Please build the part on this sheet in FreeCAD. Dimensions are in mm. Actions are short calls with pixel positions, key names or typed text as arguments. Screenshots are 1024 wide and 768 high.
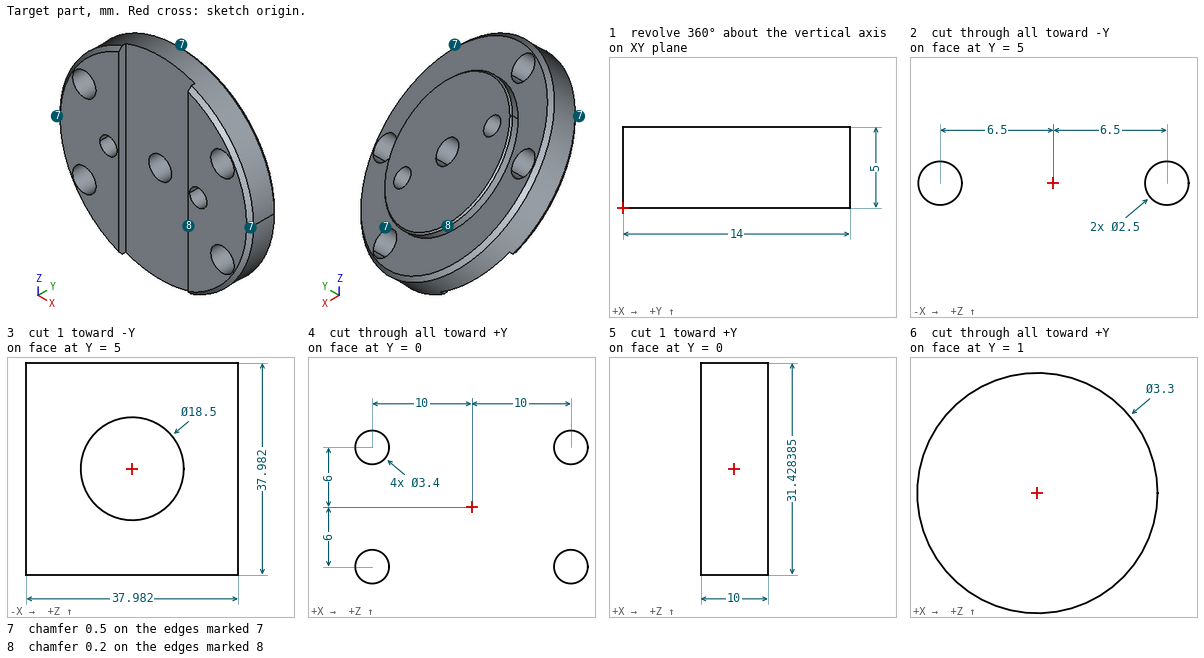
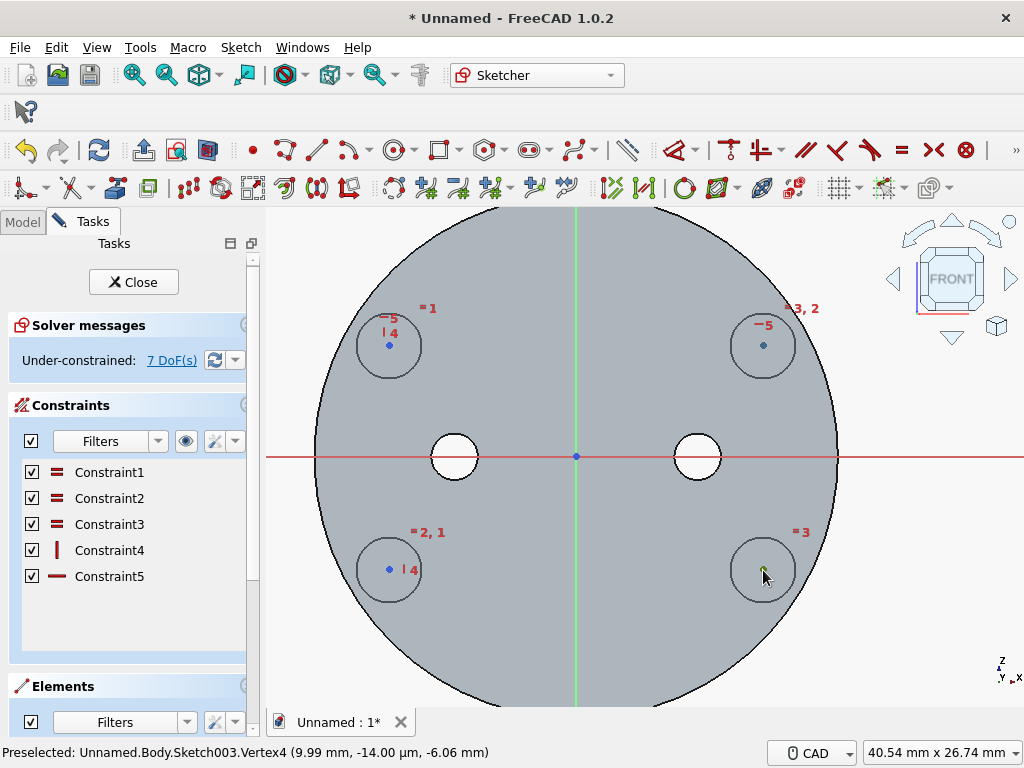
click(784, 150)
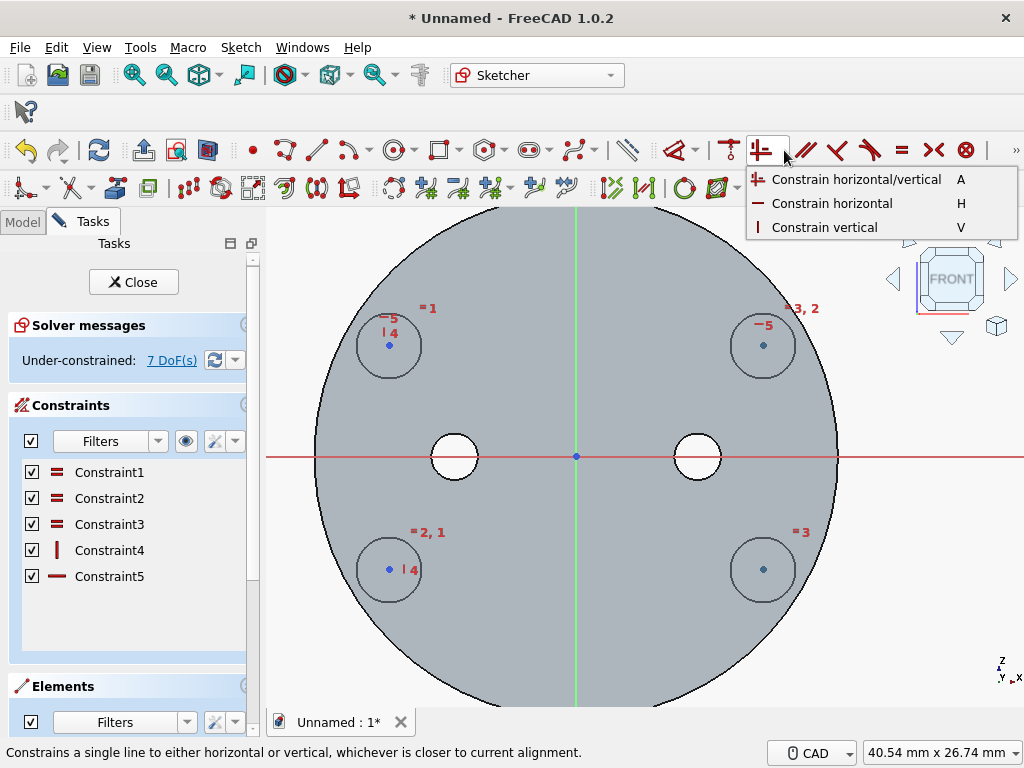
click(882, 227)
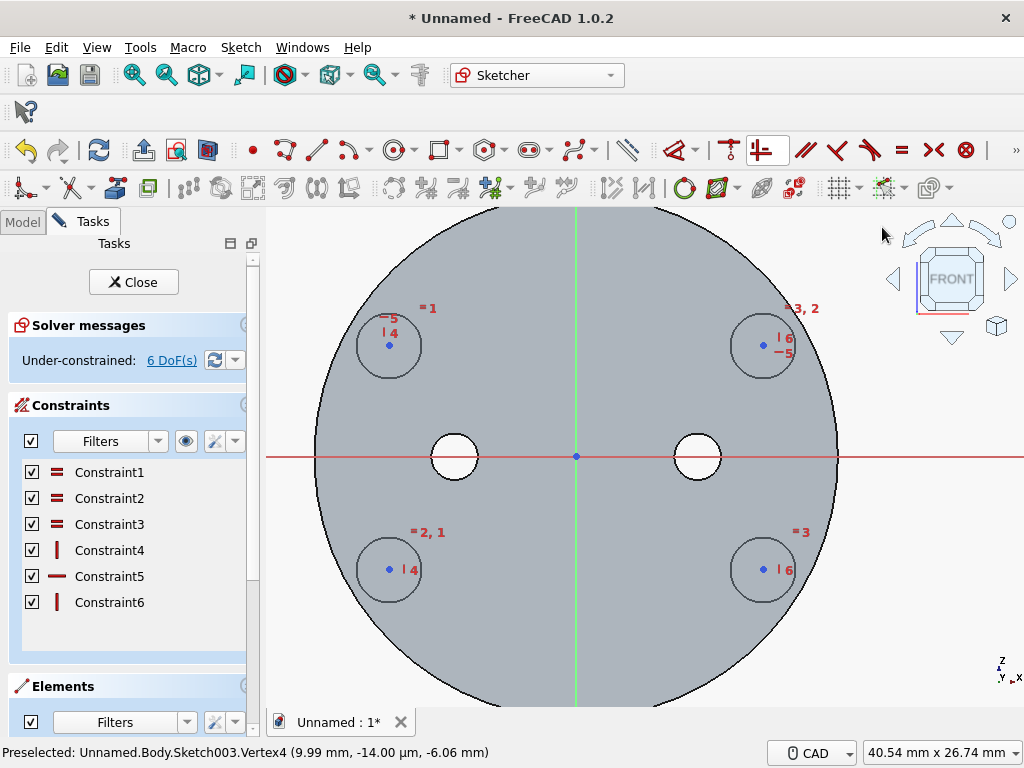
click(389, 570)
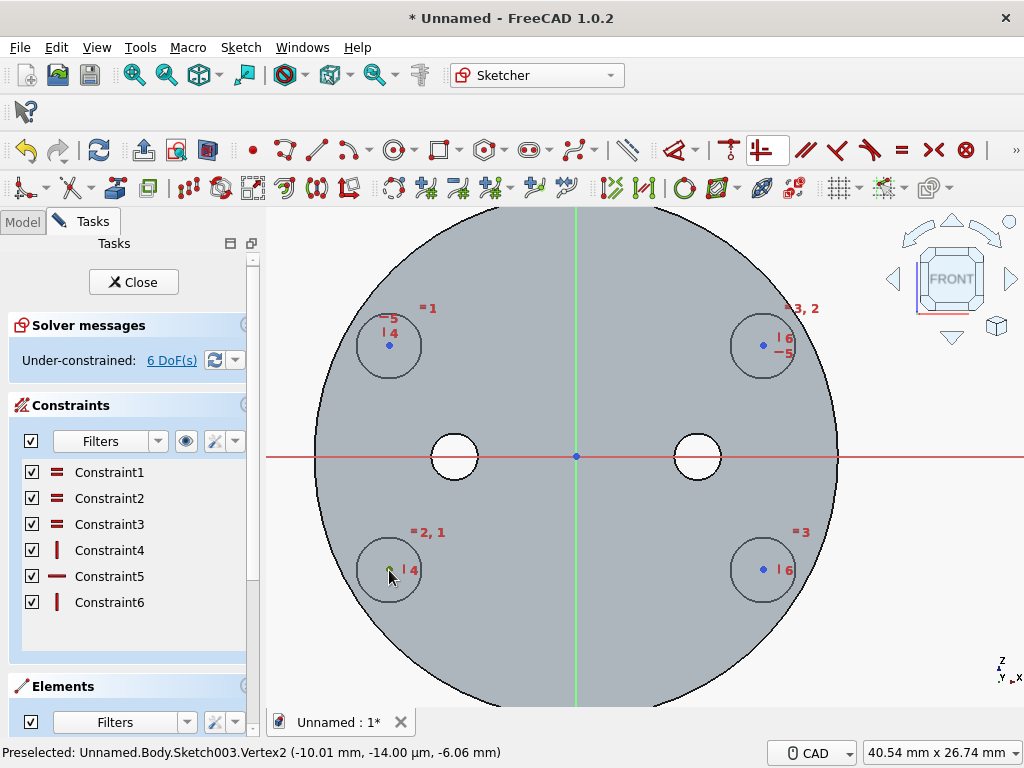
click(763, 570)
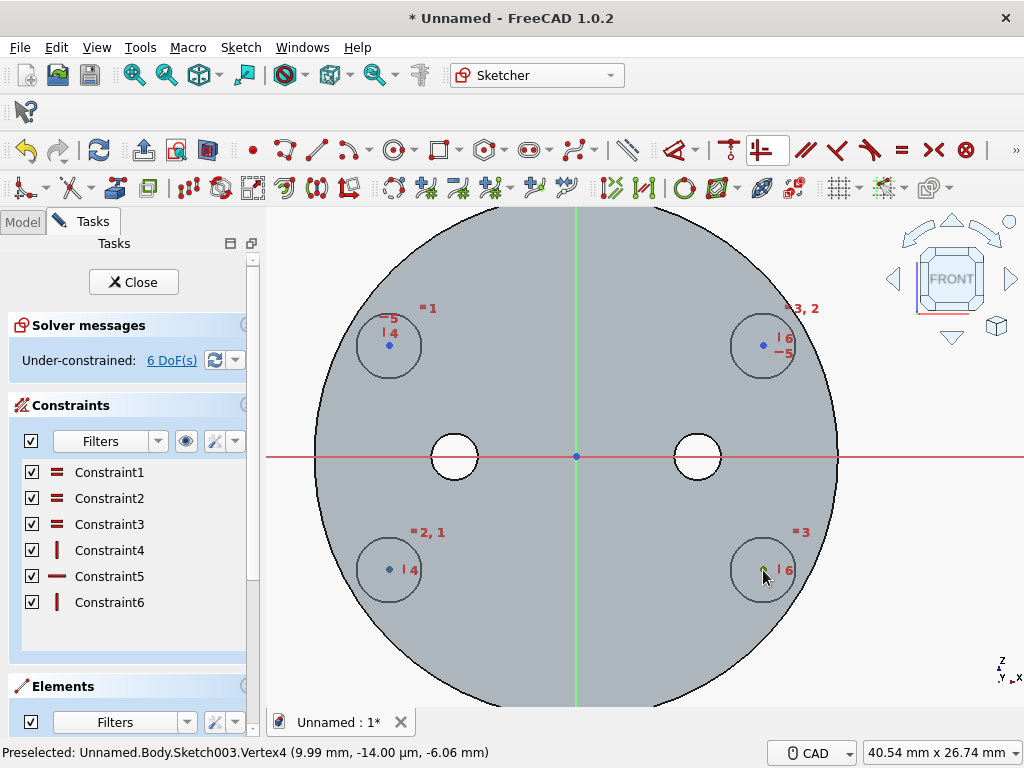
key(h)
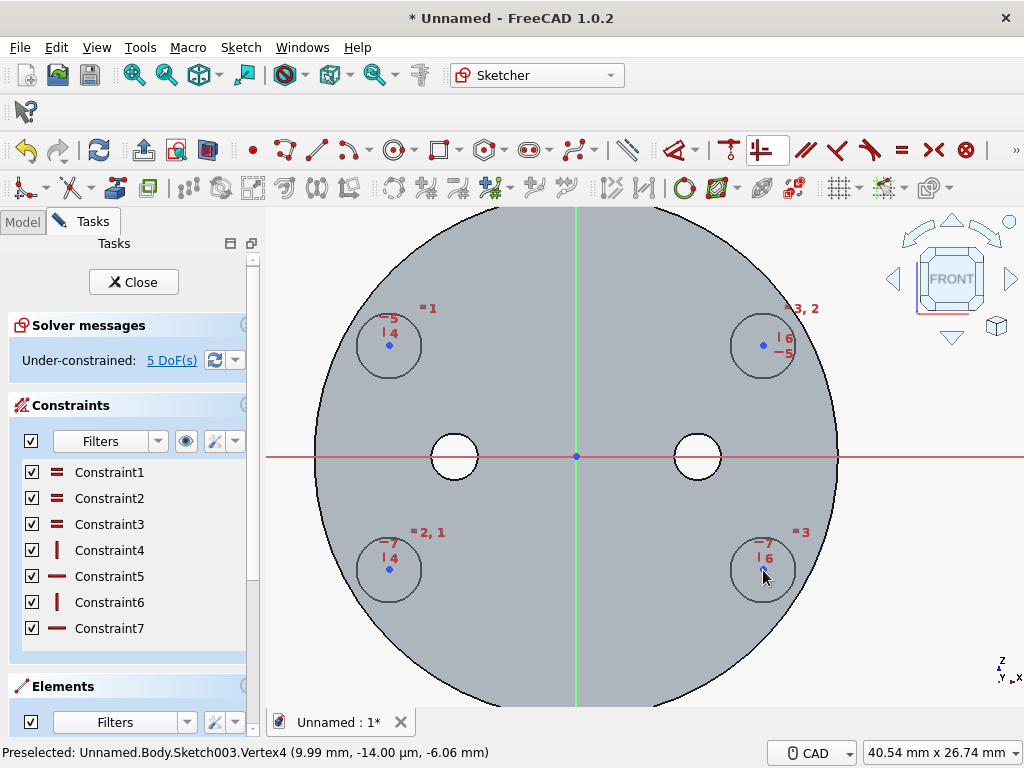
click(674, 150)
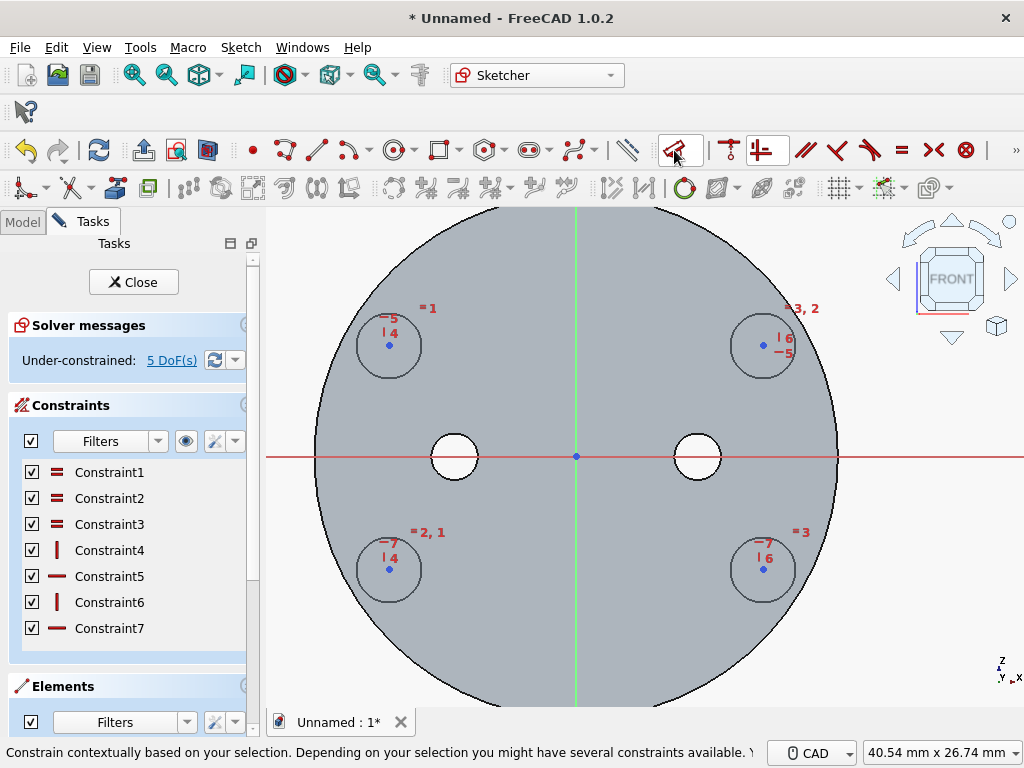
click(412, 323)
click(435, 300)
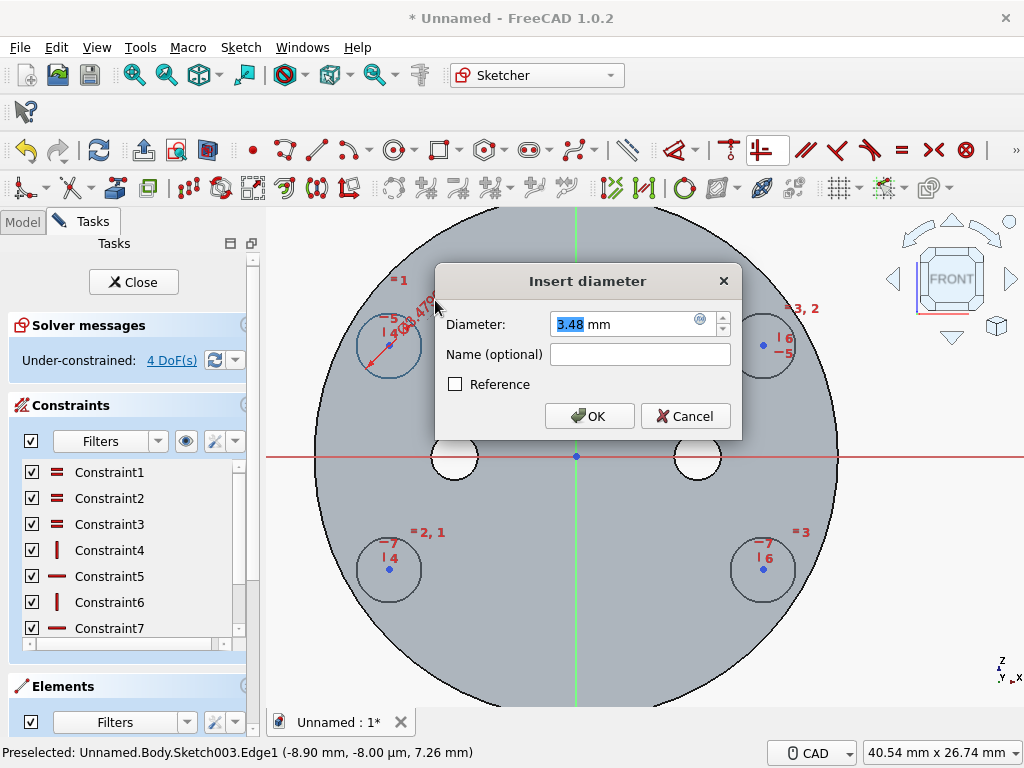
text(3.4)
key(Return)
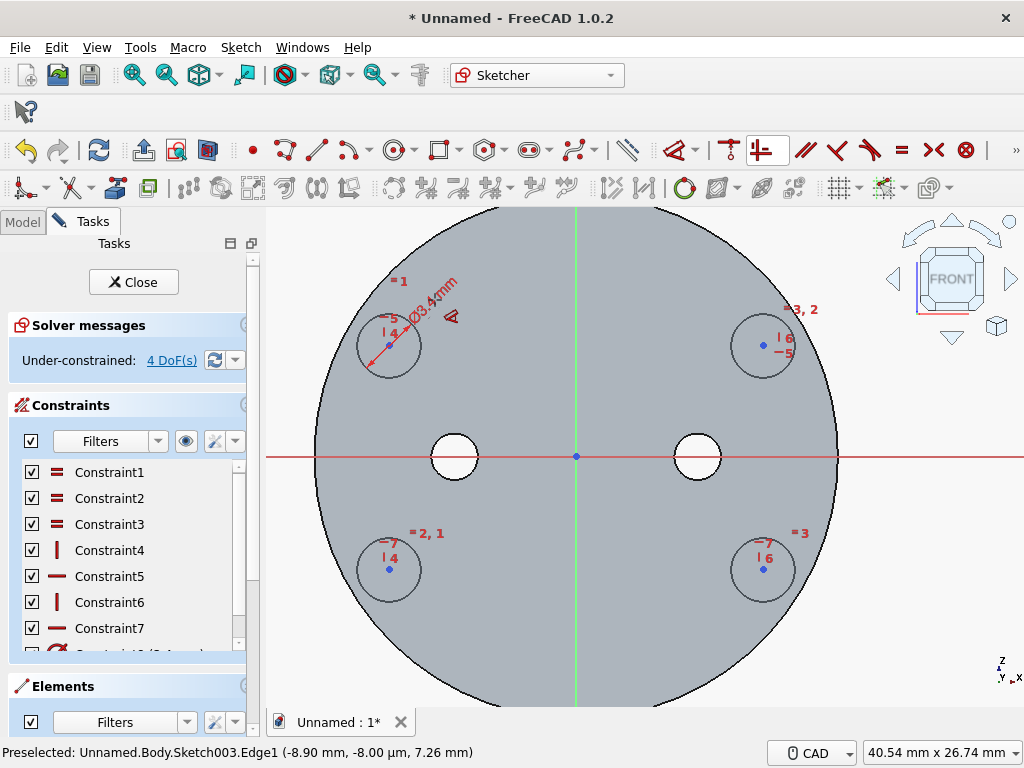
click(389, 346)
click(355, 401)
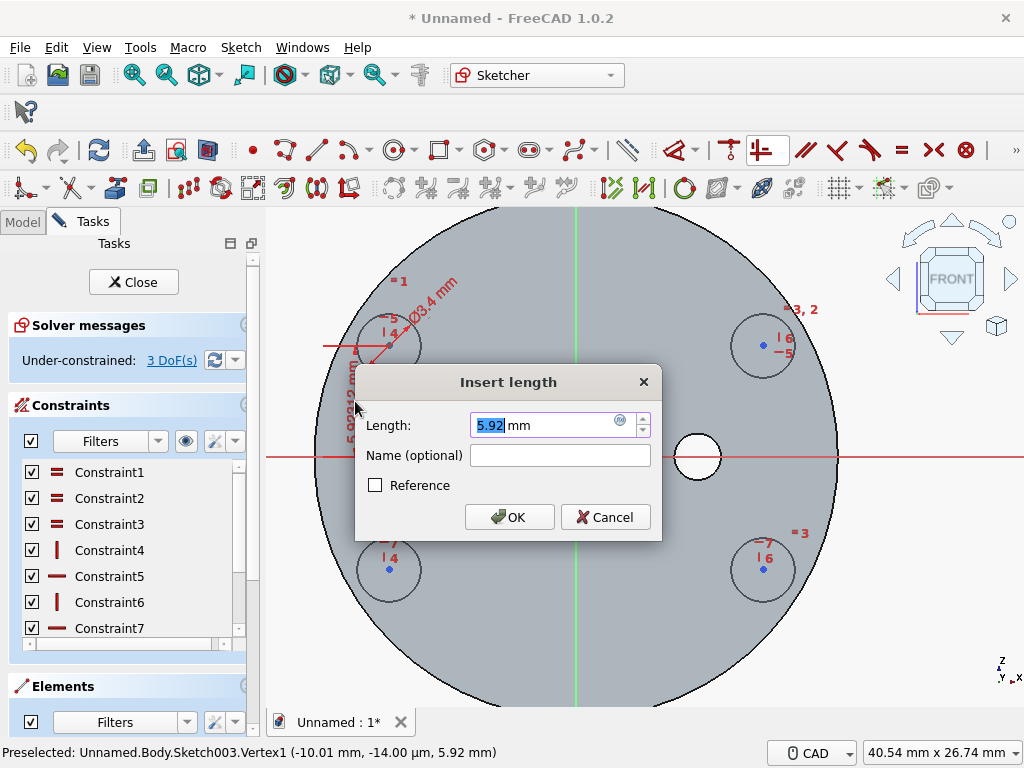
text(6)
key(Return)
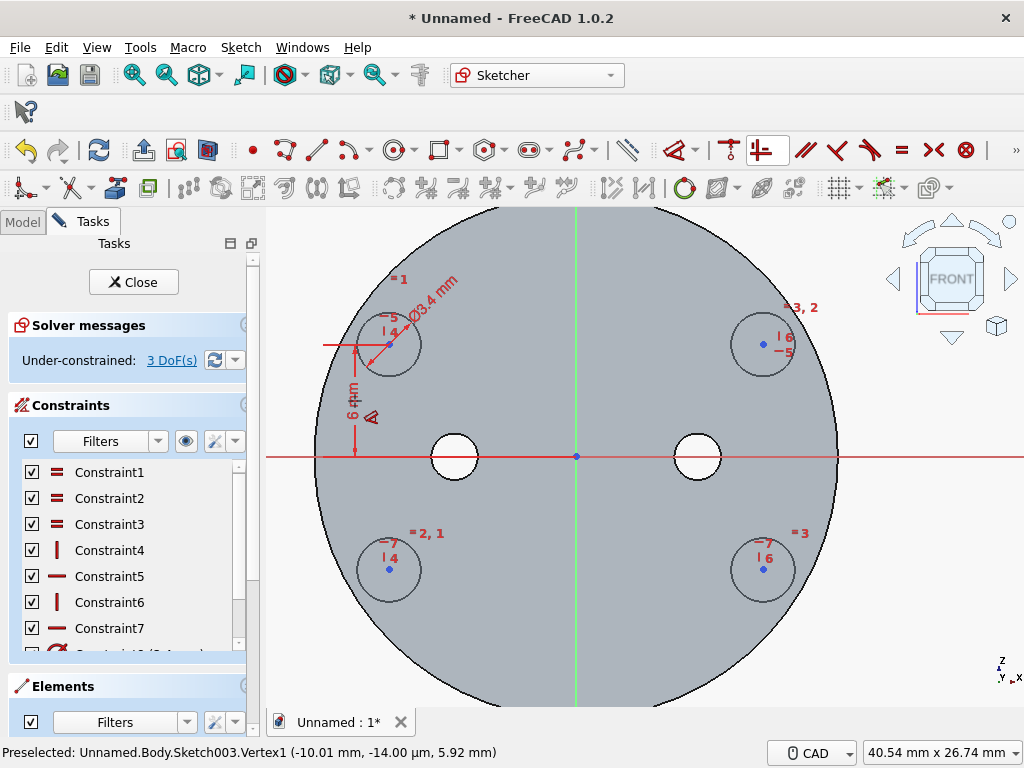
click(389, 570)
click(355, 513)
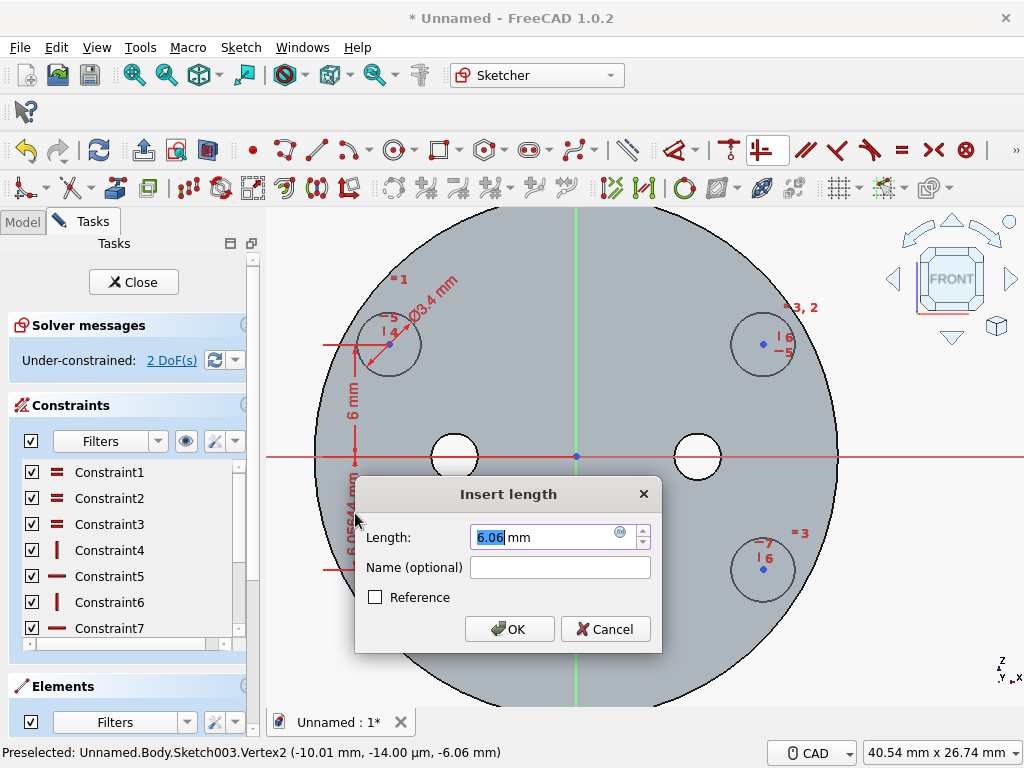
text(6)
key(Return)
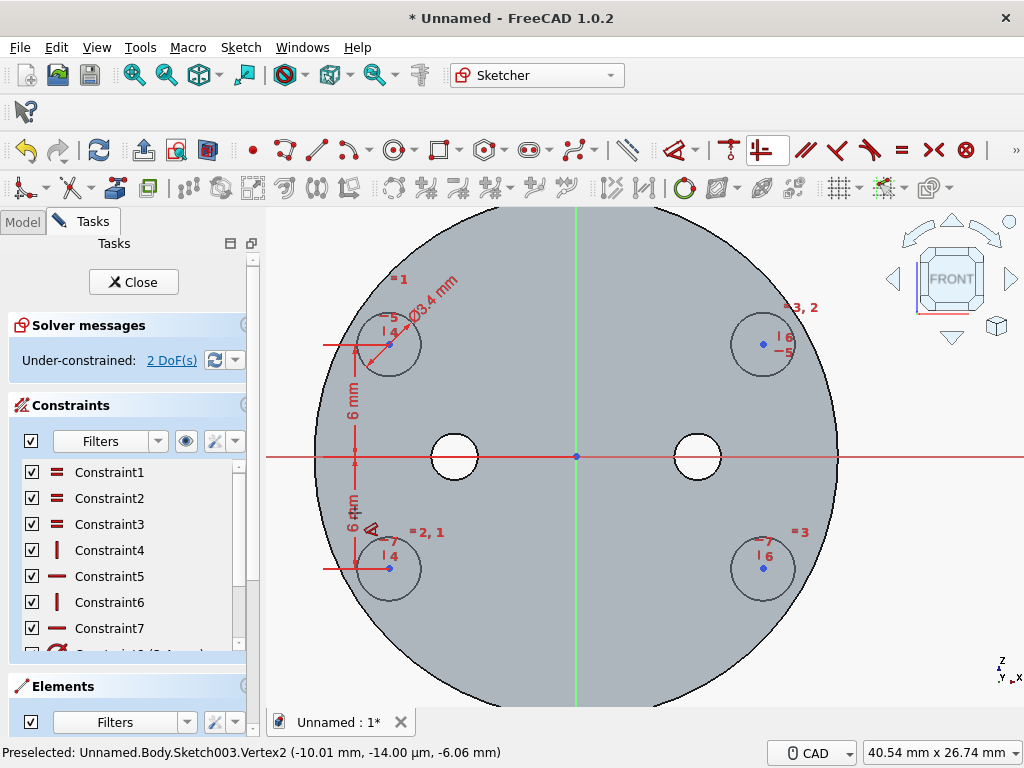
click(389, 345)
click(526, 311)